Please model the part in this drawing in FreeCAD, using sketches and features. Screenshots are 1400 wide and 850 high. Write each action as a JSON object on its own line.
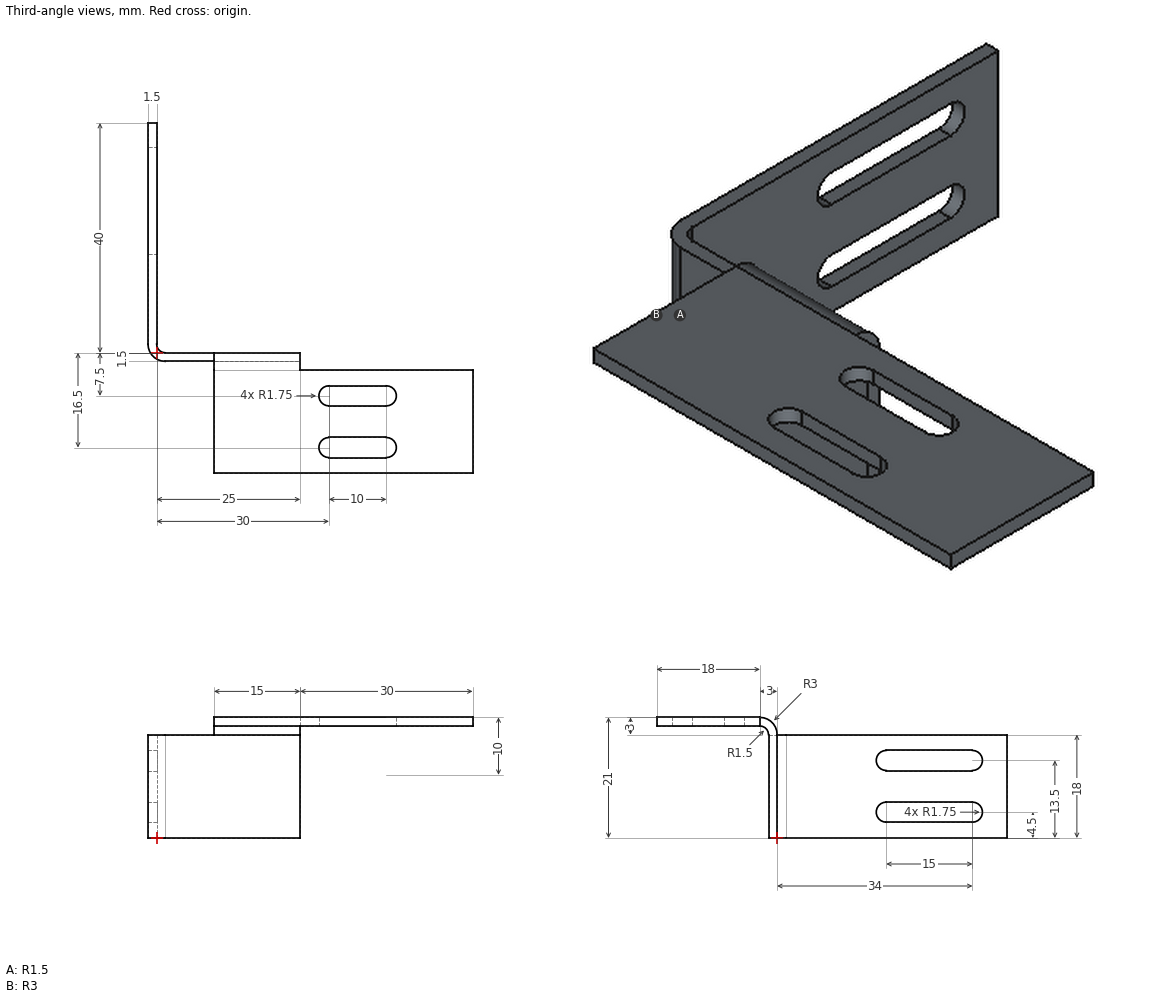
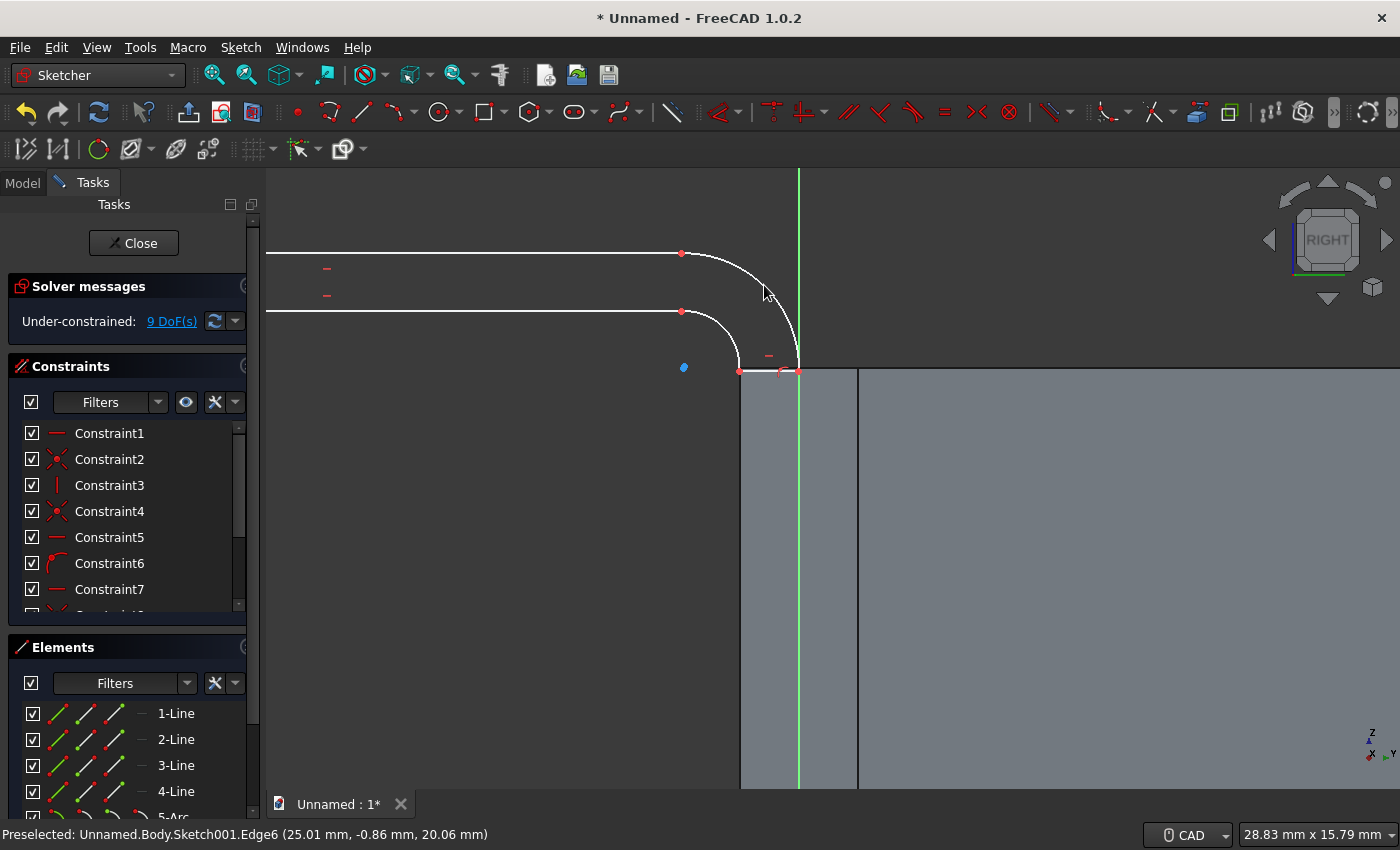
{"action": "left_click", "coordinate": [469, 253]}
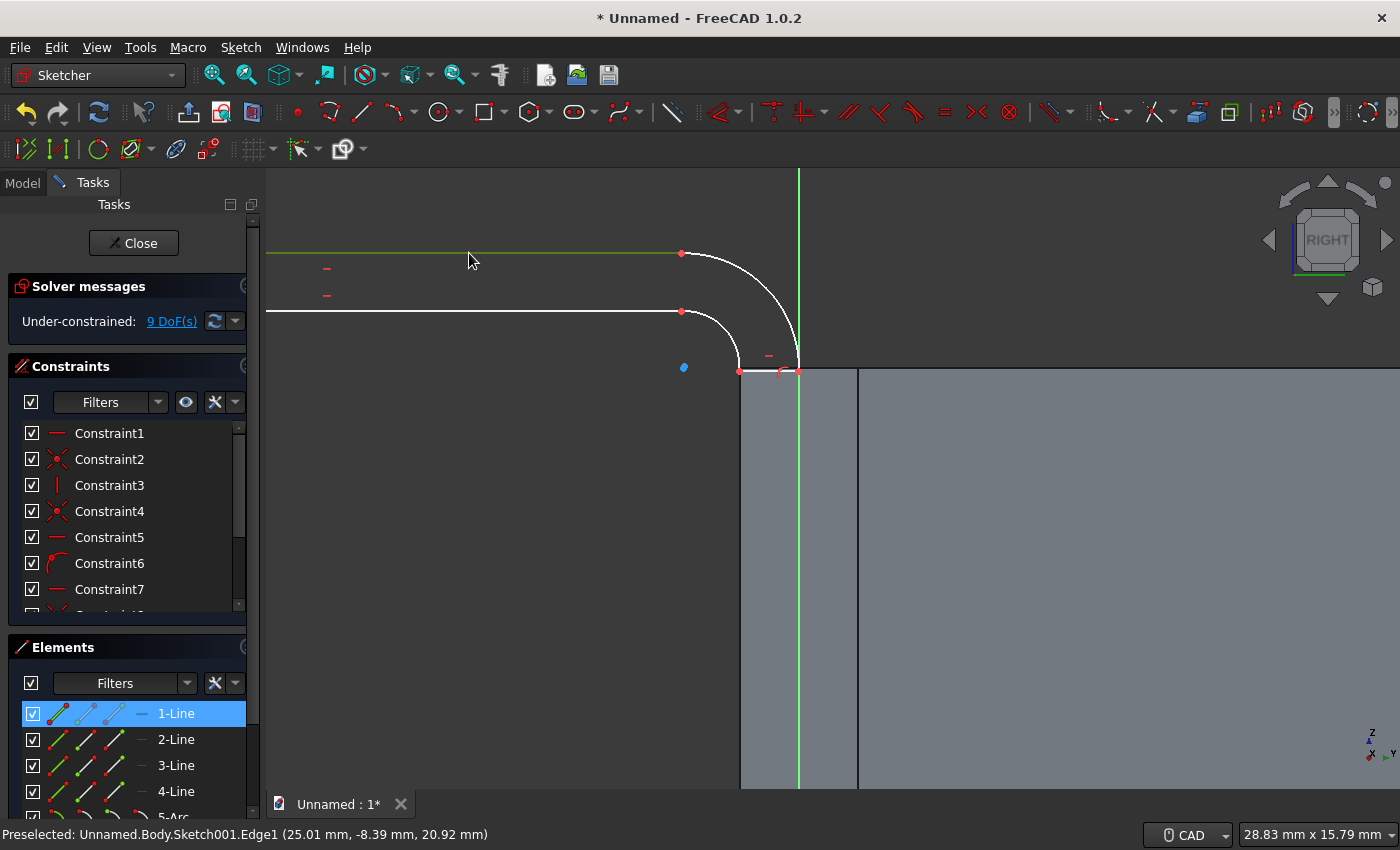
{"action": "left_click", "coordinate": [787, 317]}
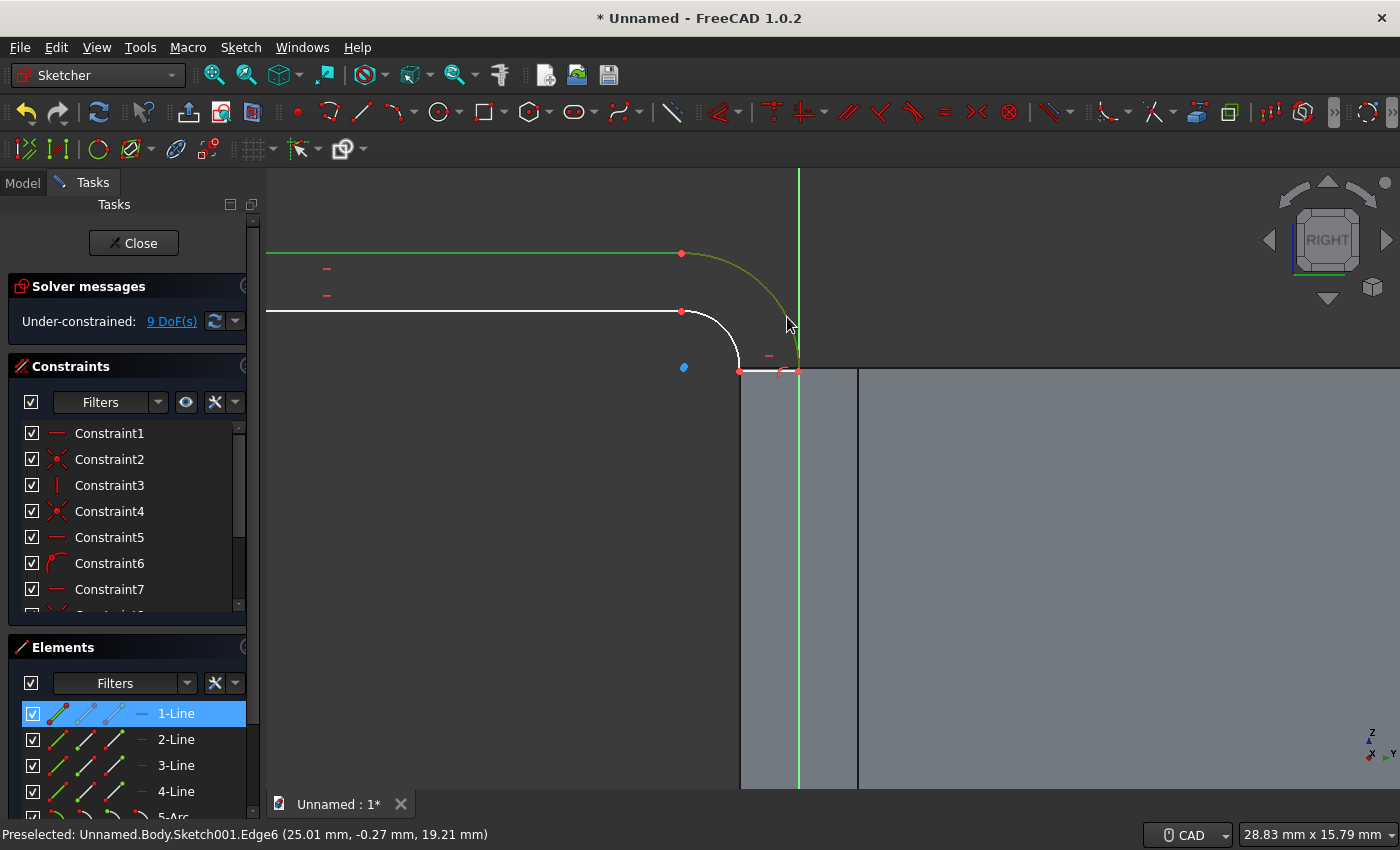
{"action": "key", "text": "t"}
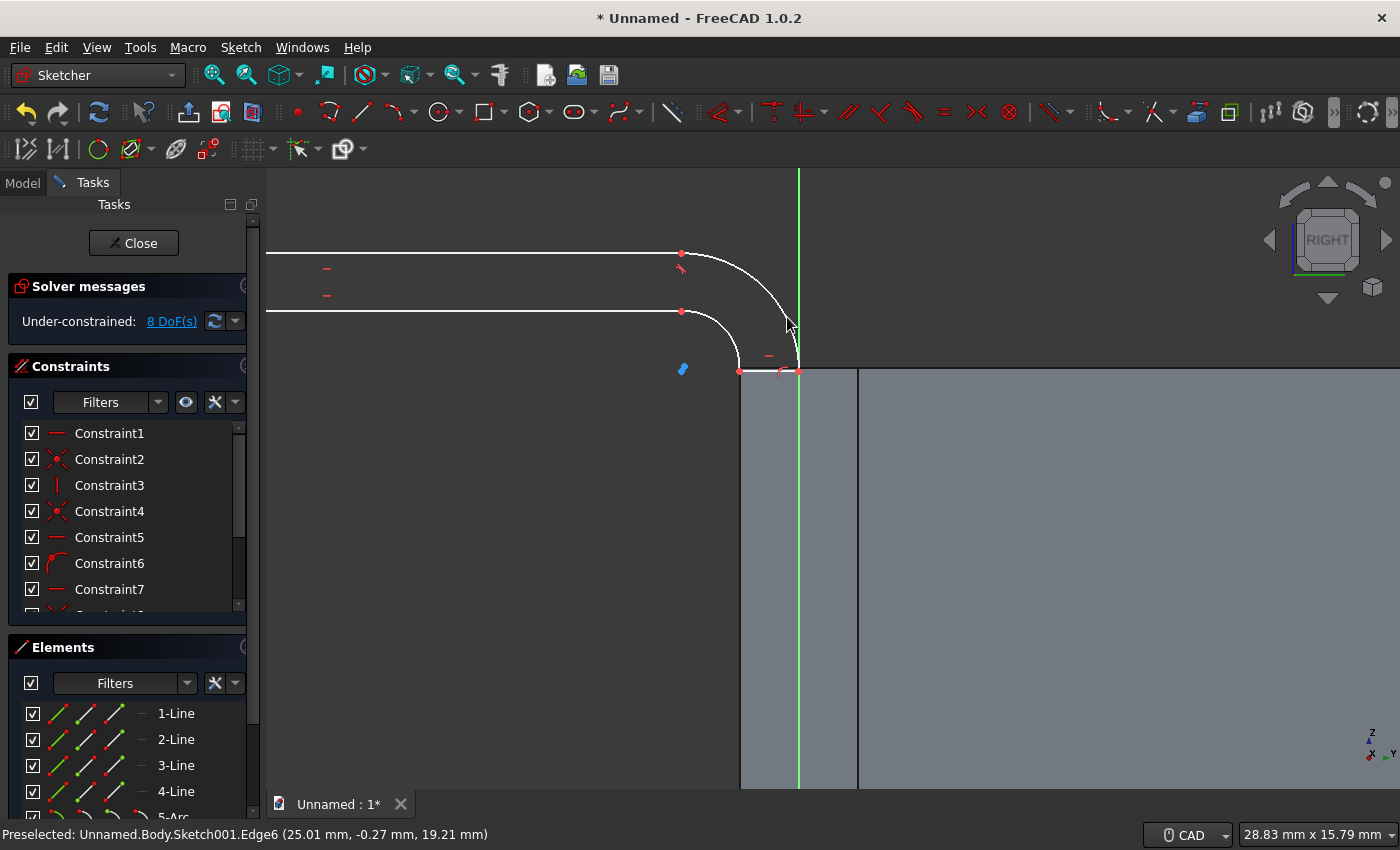
{"action": "left_click", "coordinate": [469, 311]}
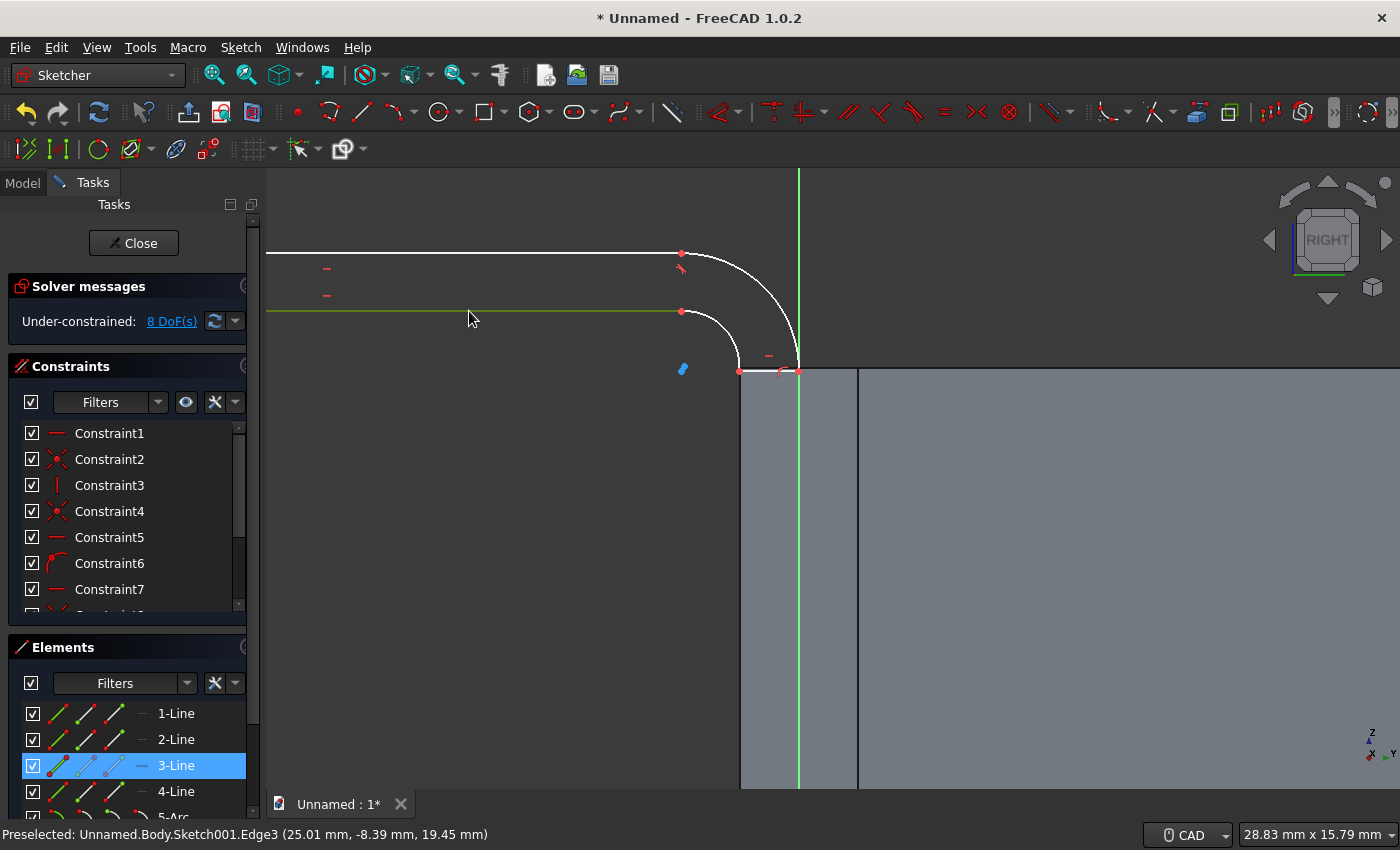
{"action": "left_click", "coordinate": [734, 344]}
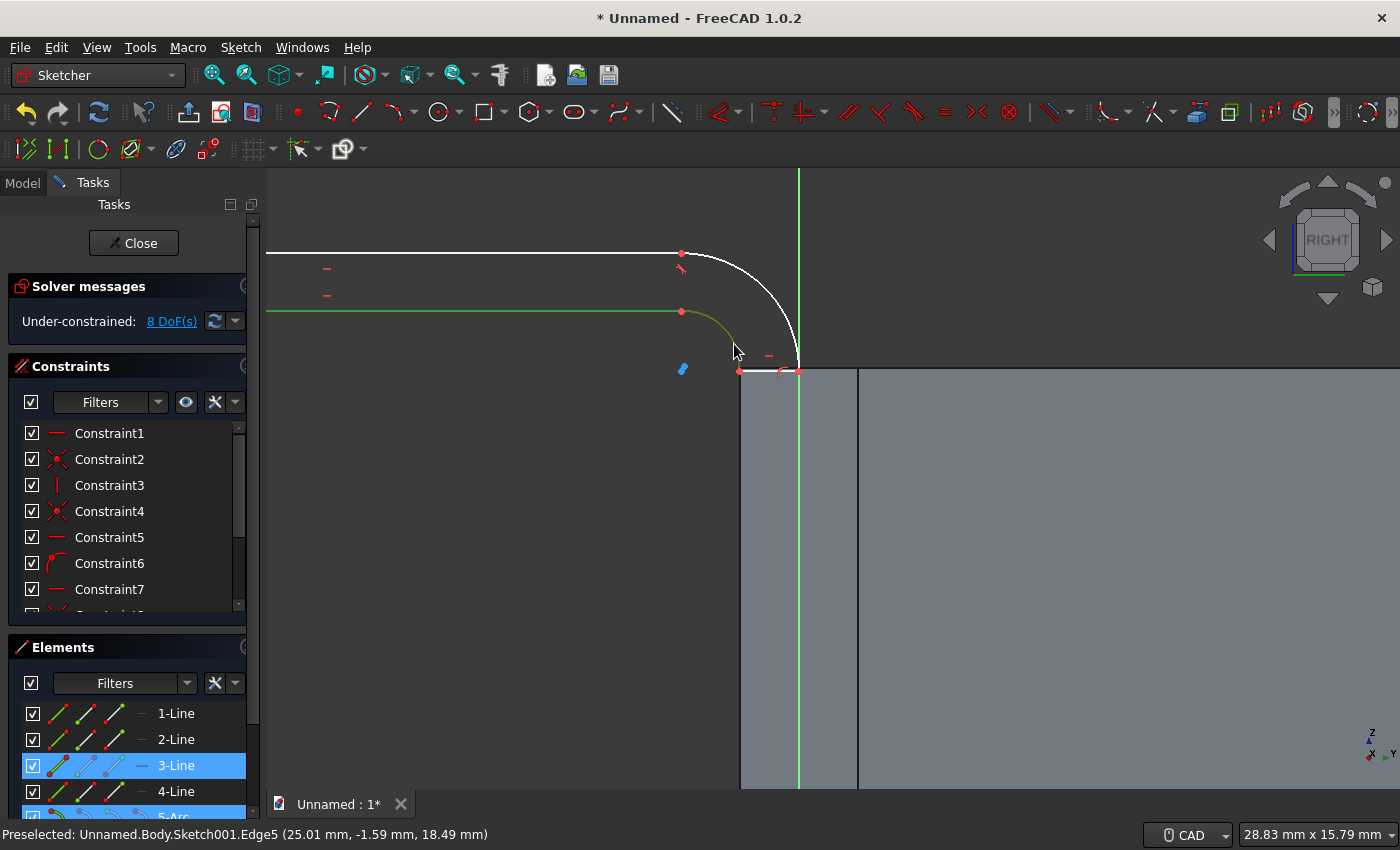
{"action": "left_click", "coordinate": [914, 112]}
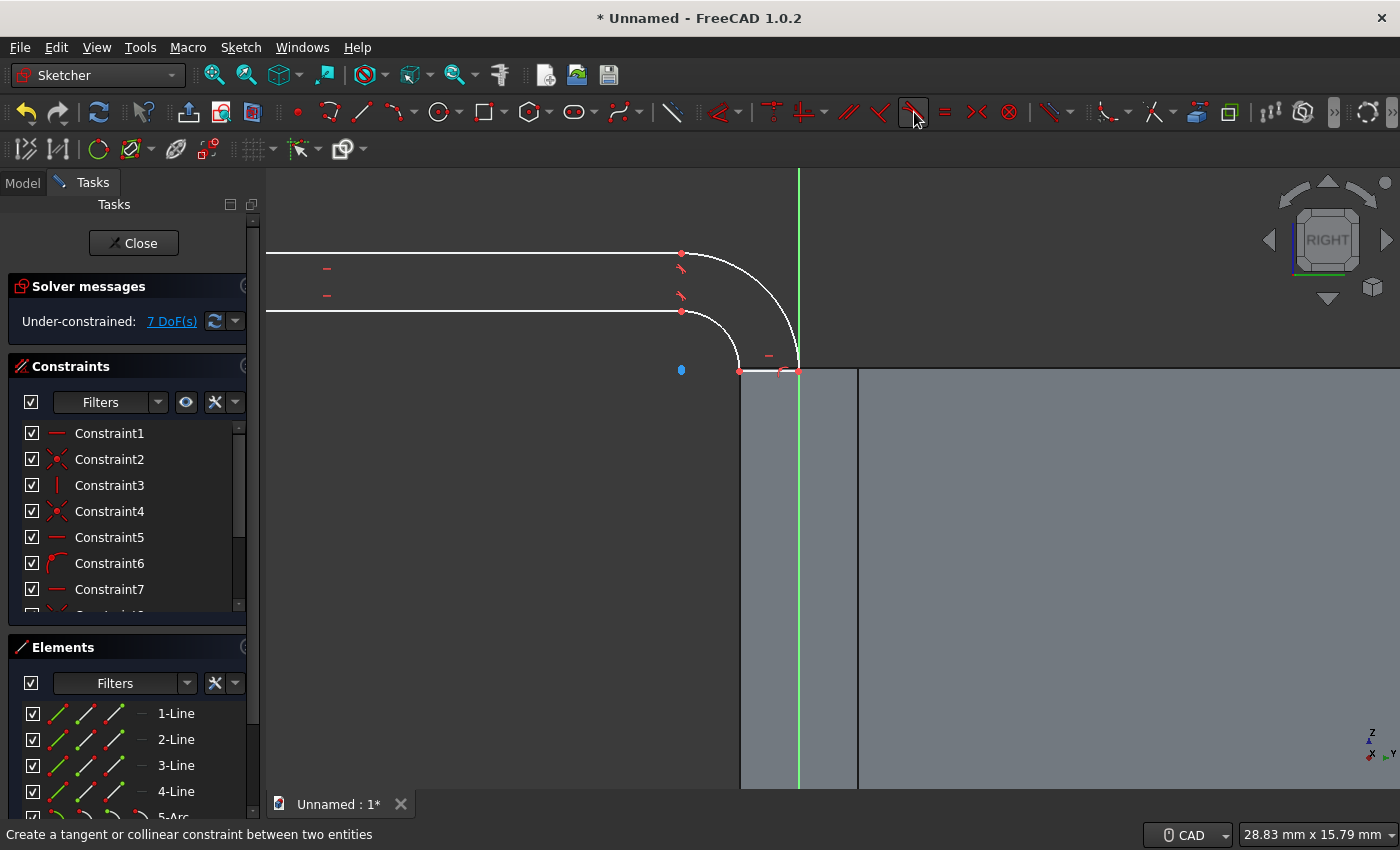
{"action": "left_click", "coordinate": [734, 344]}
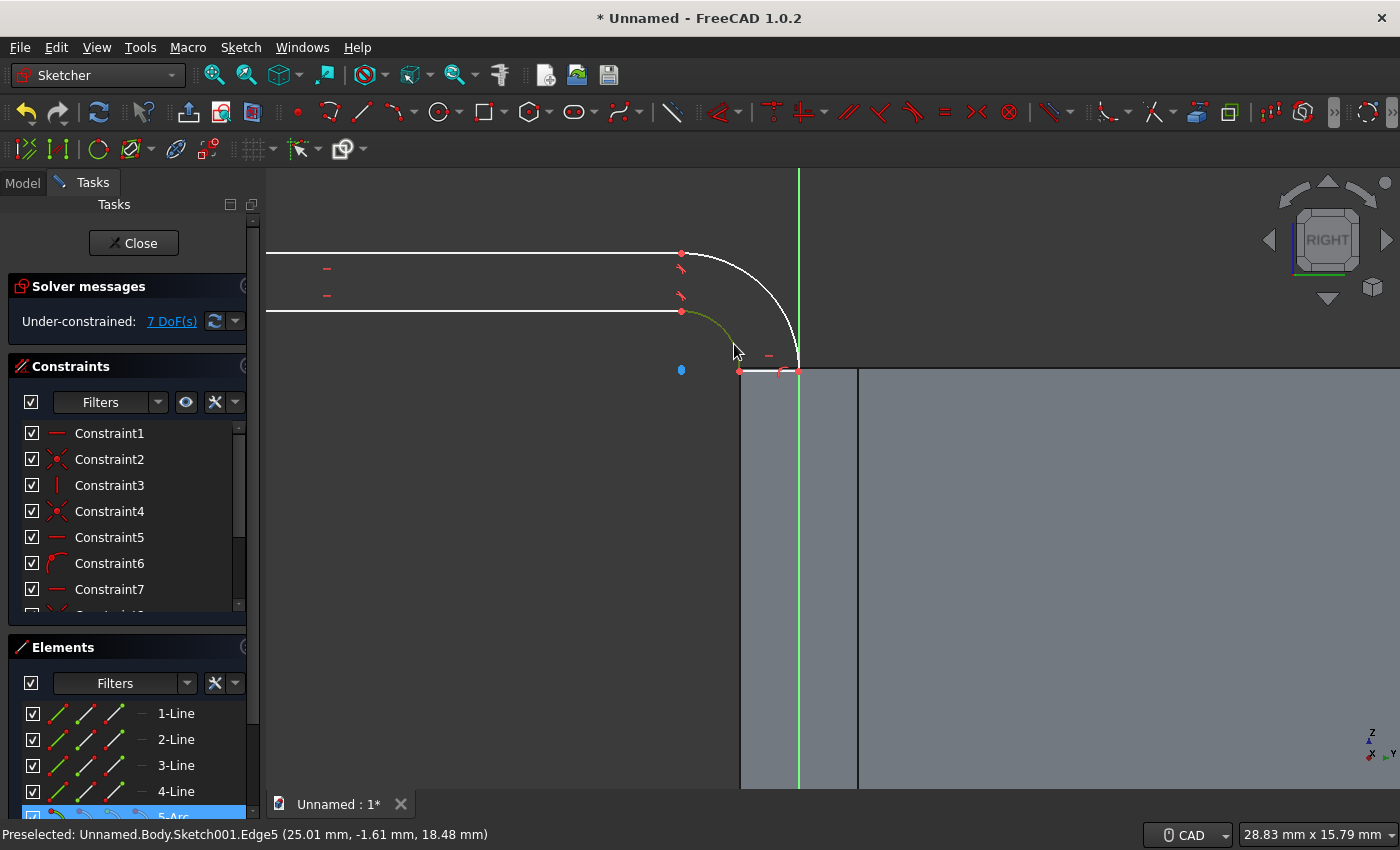
{"action": "left_click", "coordinate": [786, 318]}